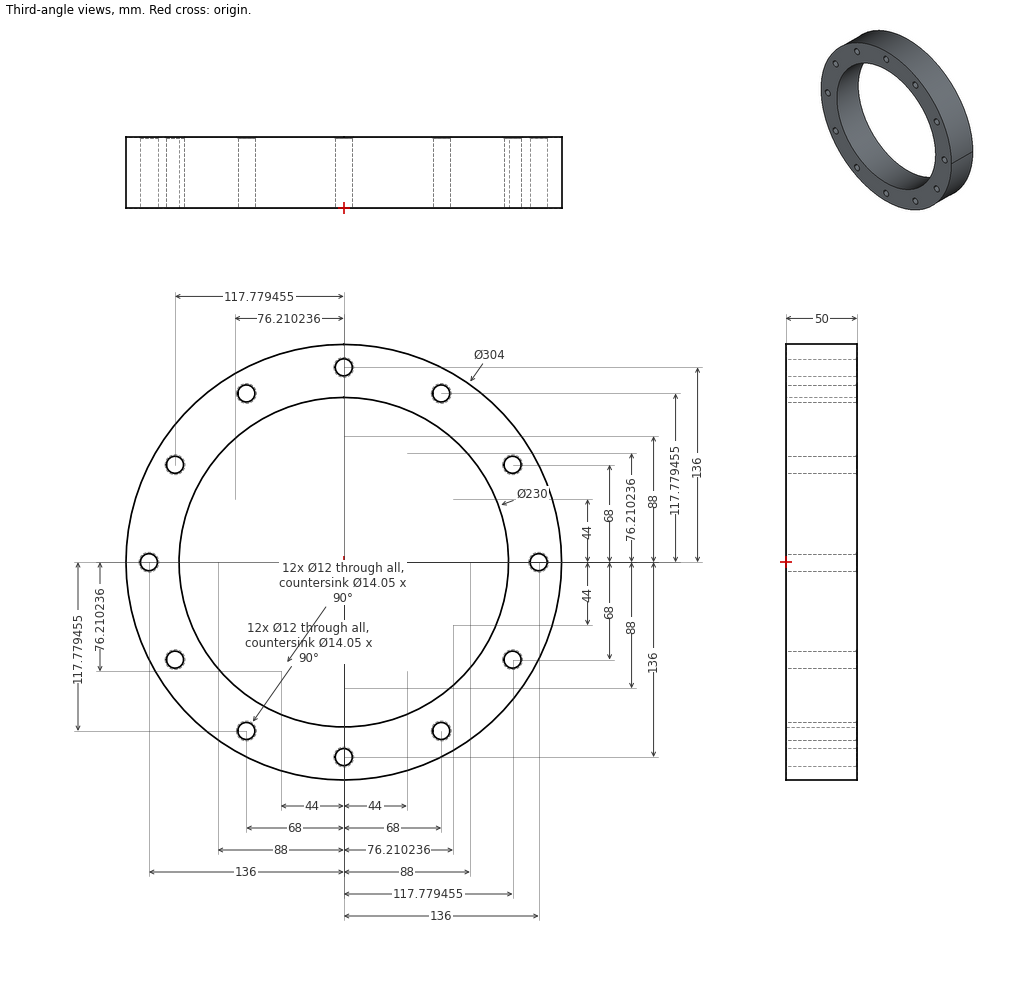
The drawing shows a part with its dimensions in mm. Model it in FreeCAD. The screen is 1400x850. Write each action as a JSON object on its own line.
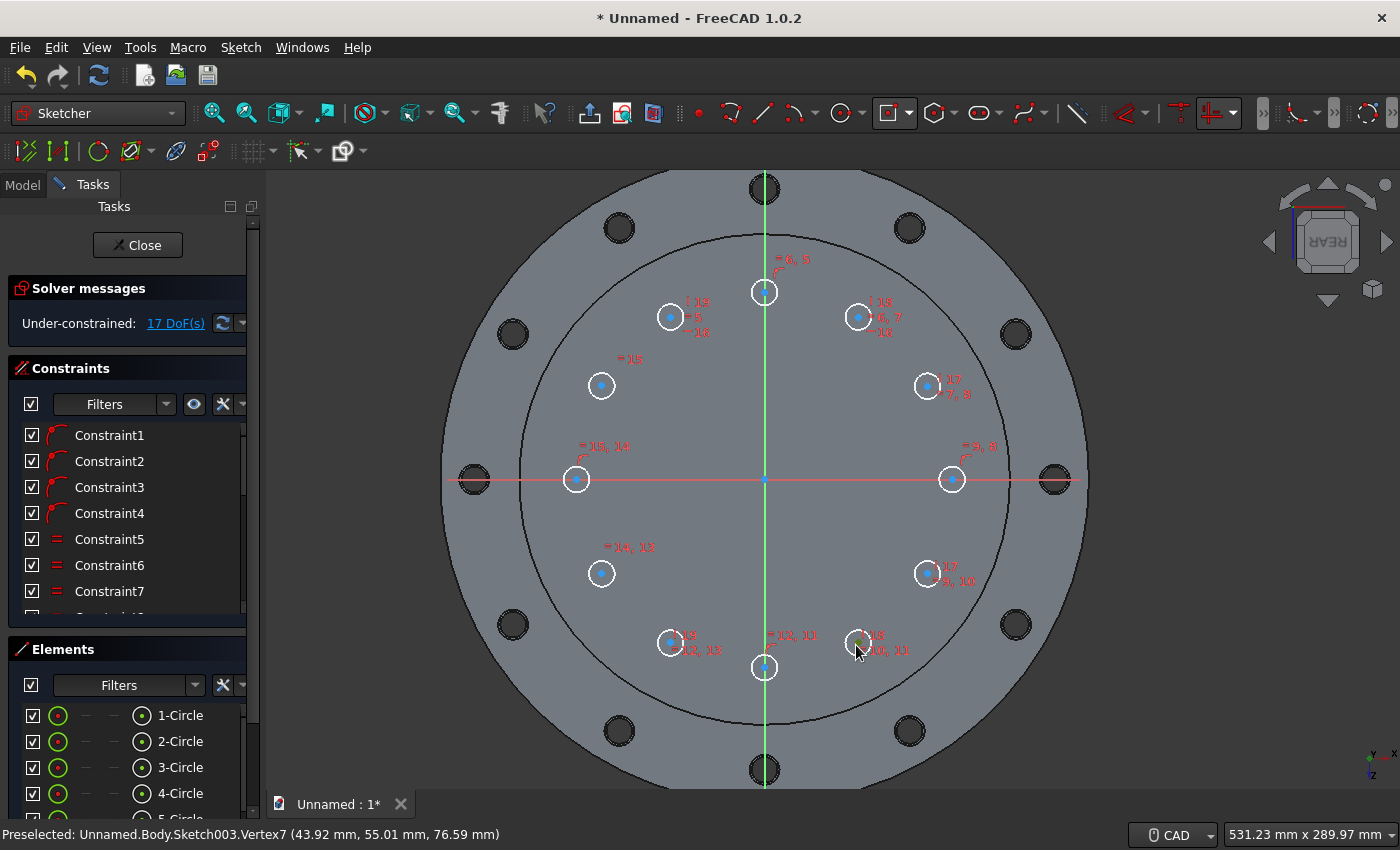
{"action": "left_click", "coordinate": [669, 645]}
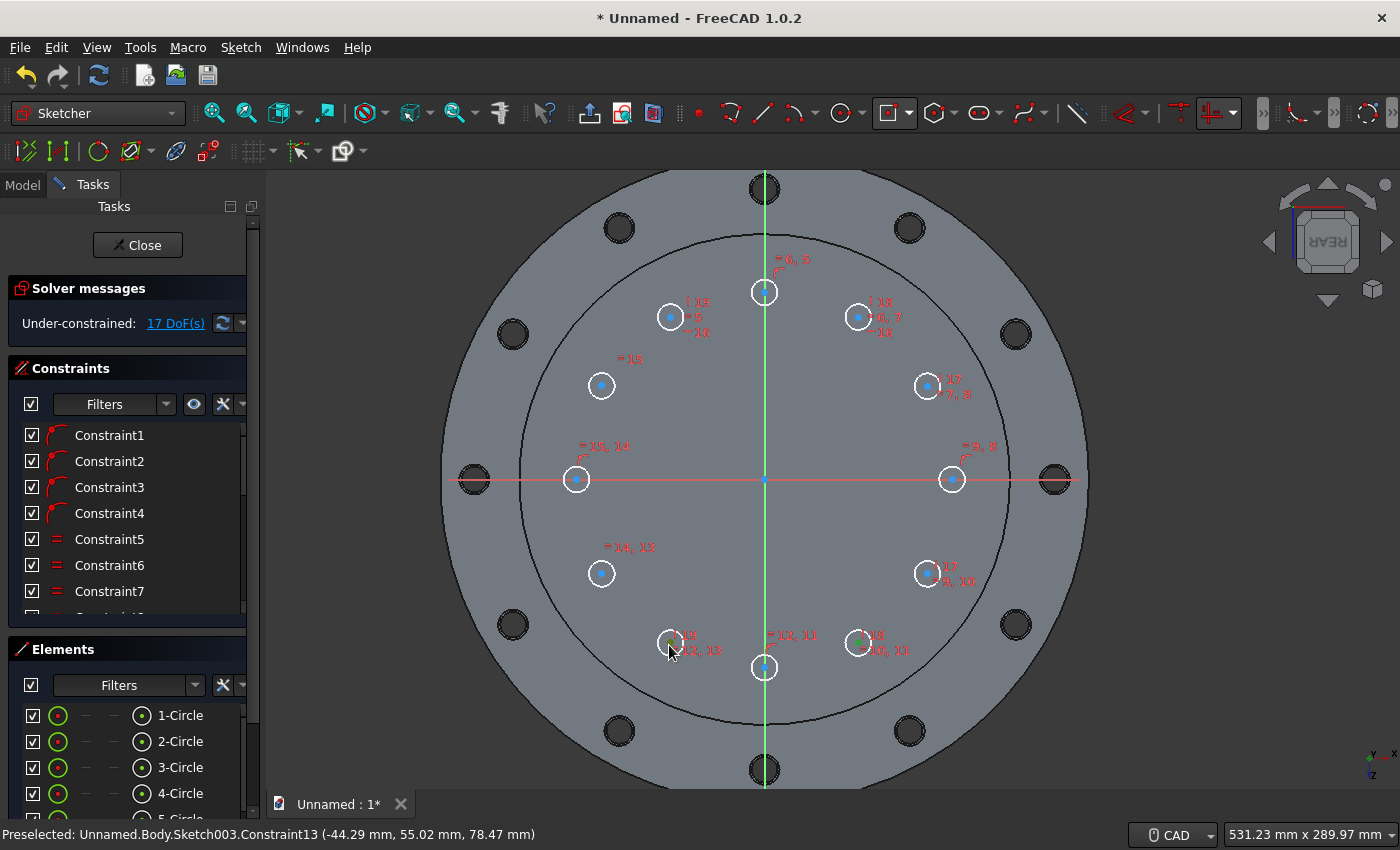
{"action": "key", "text": "h"}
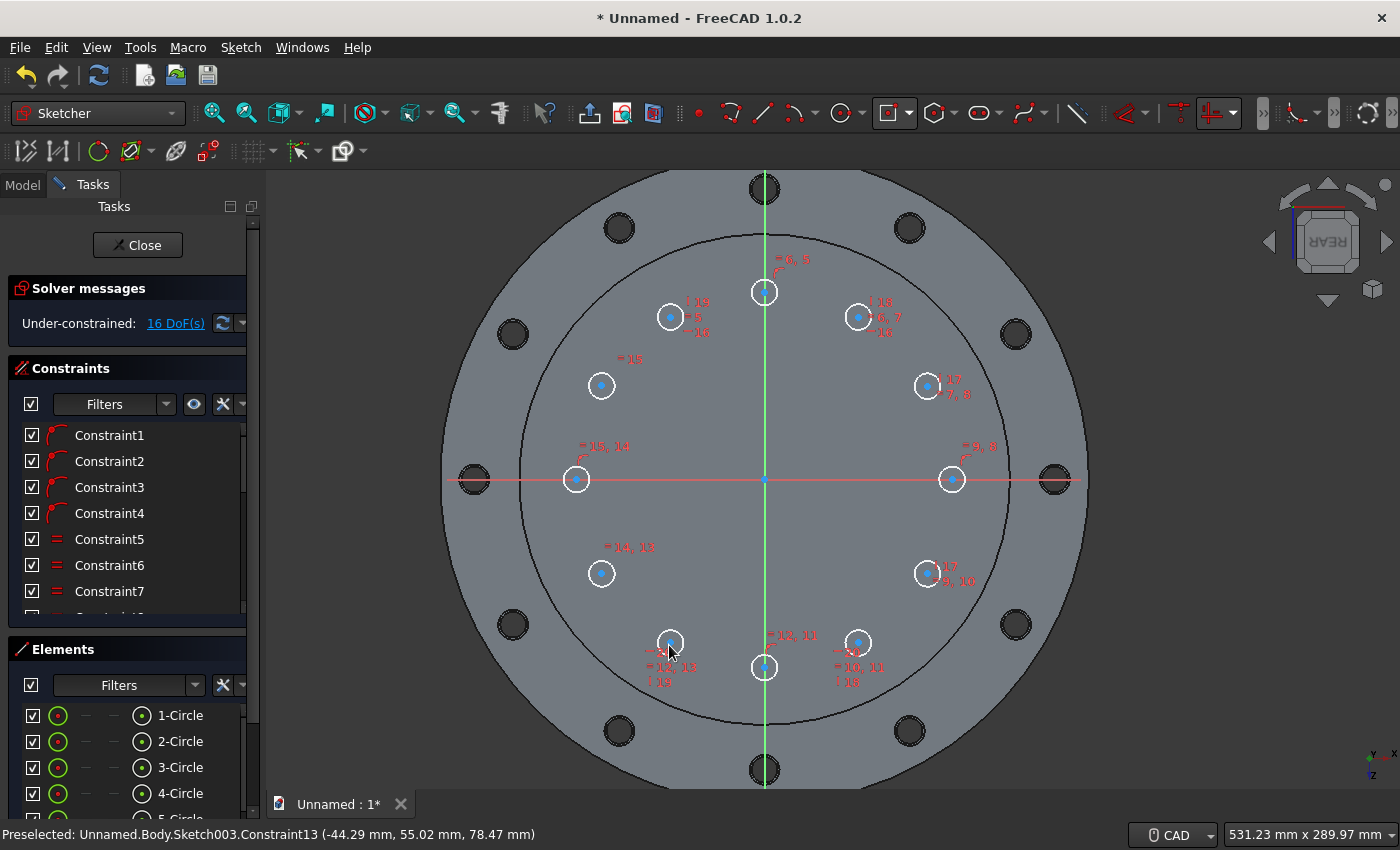
{"action": "left_click", "coordinate": [927, 574]}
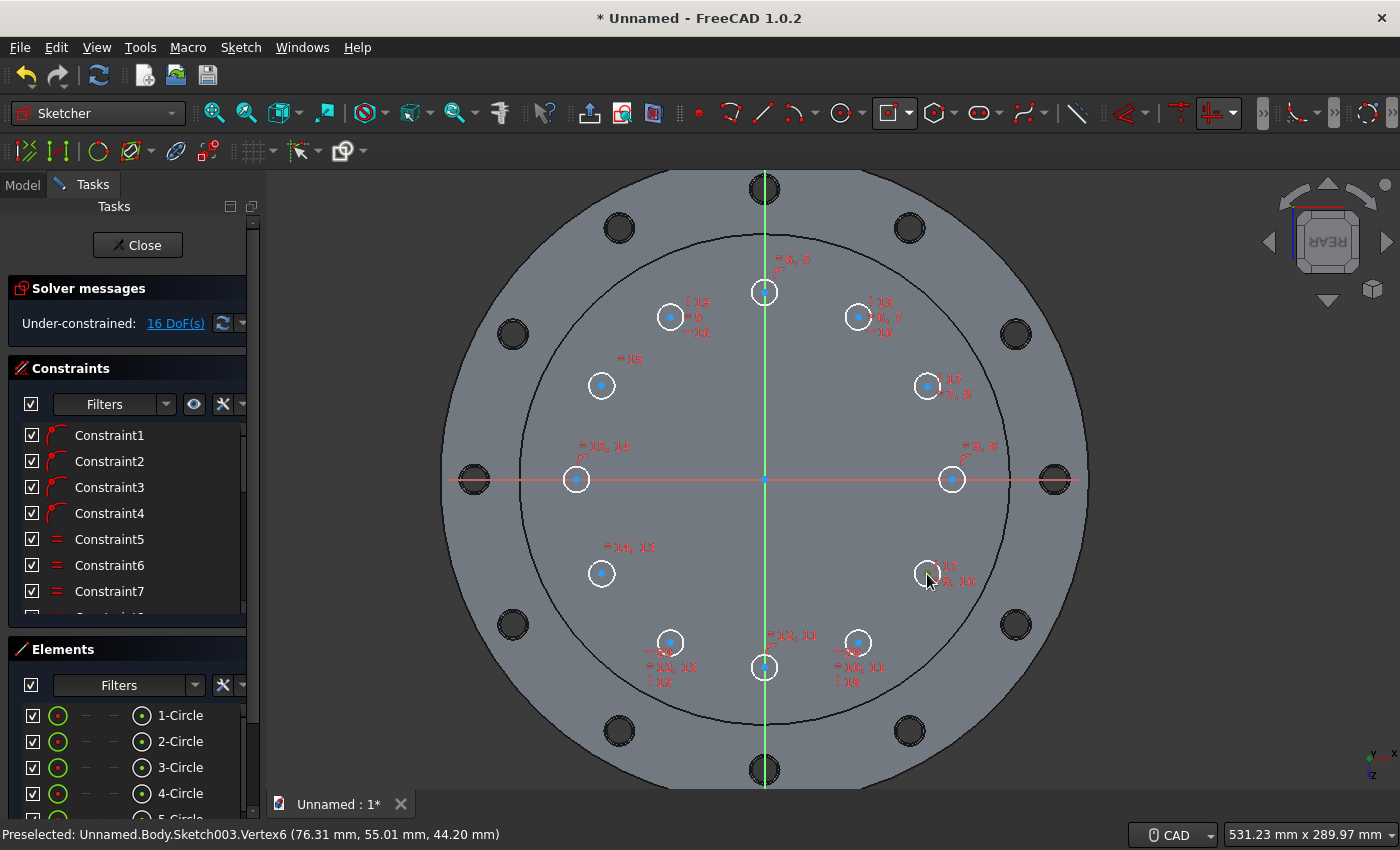
{"action": "left_click", "coordinate": [602, 574]}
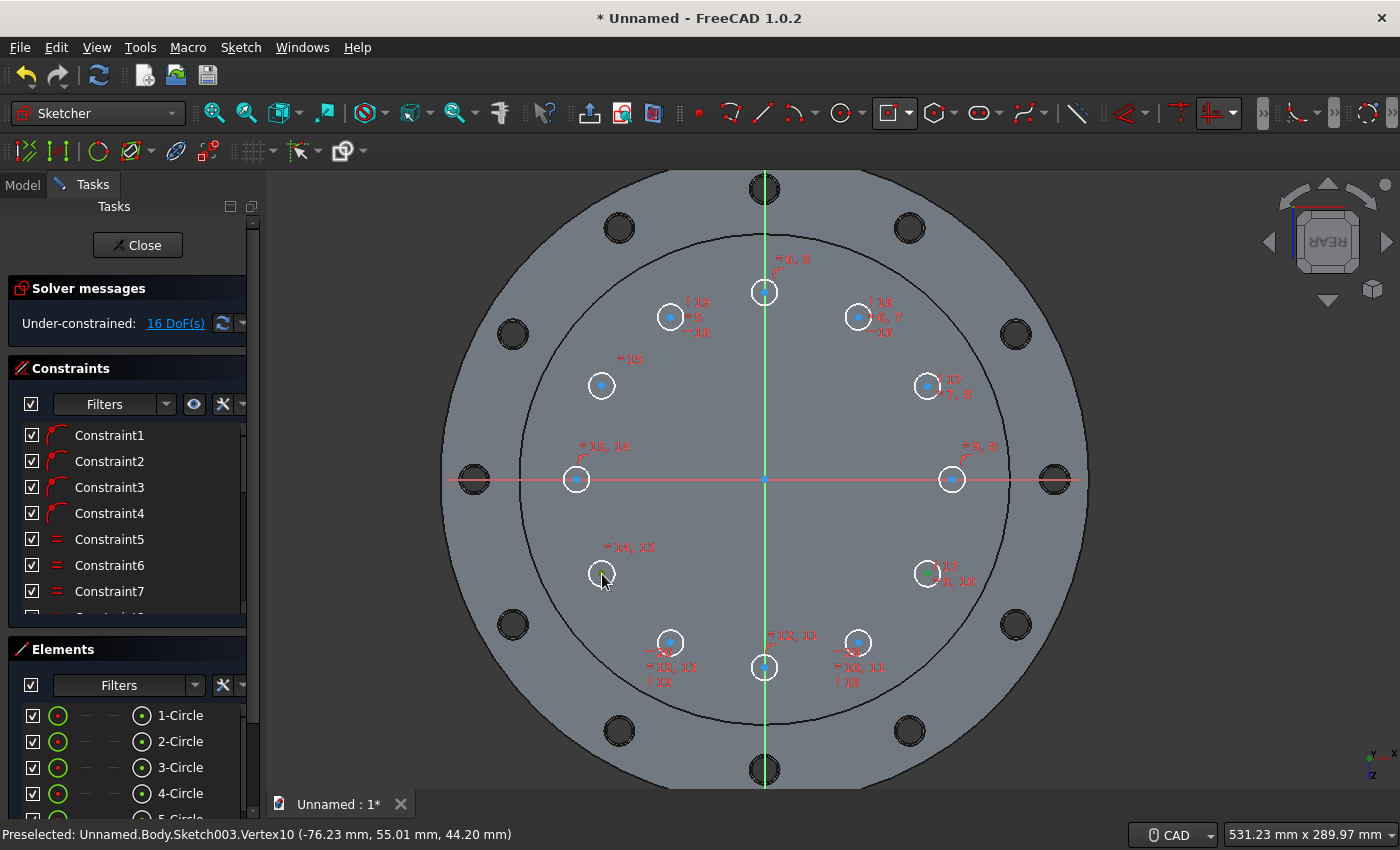
{"action": "key", "text": "h"}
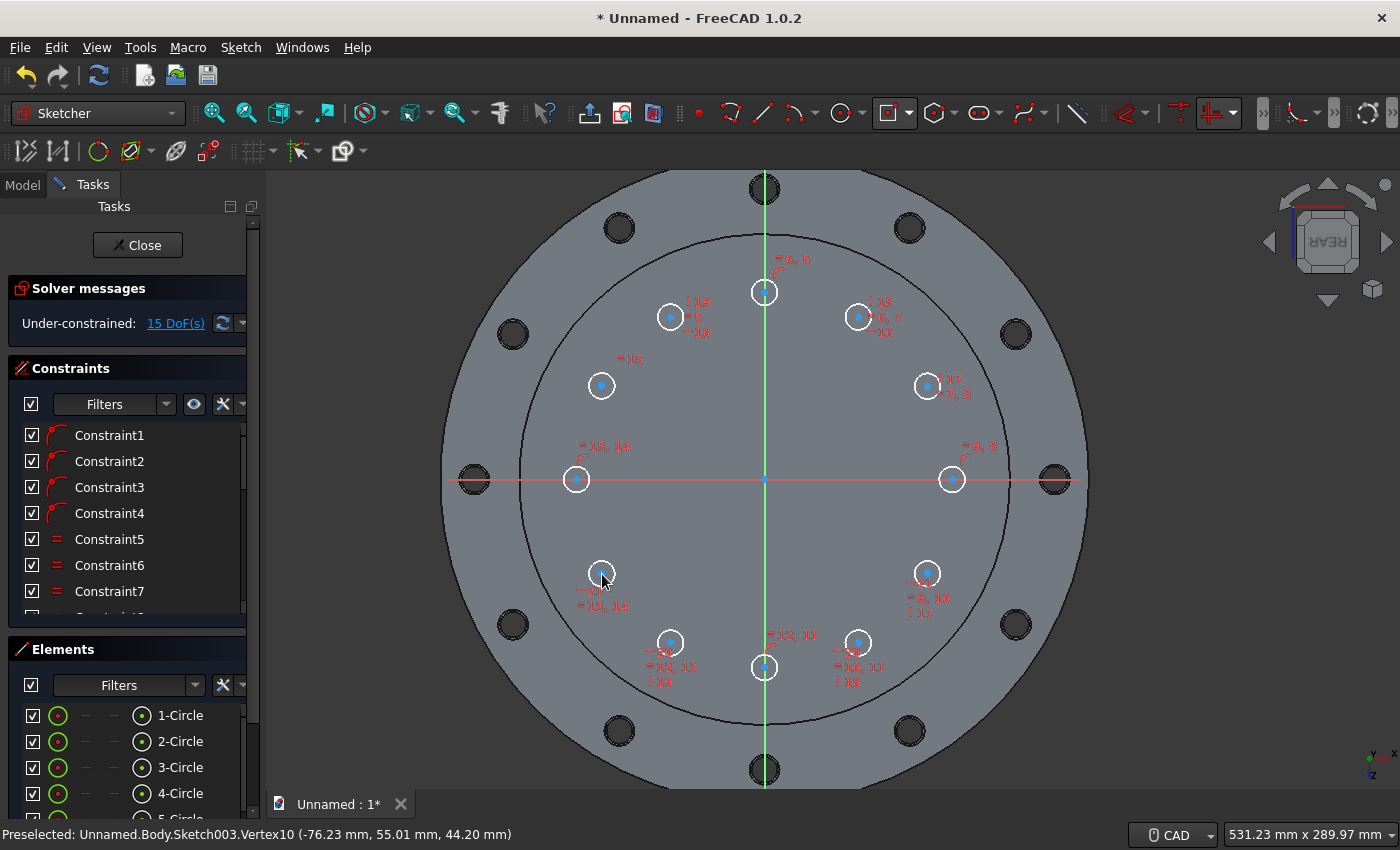
{"action": "left_click", "coordinate": [602, 574]}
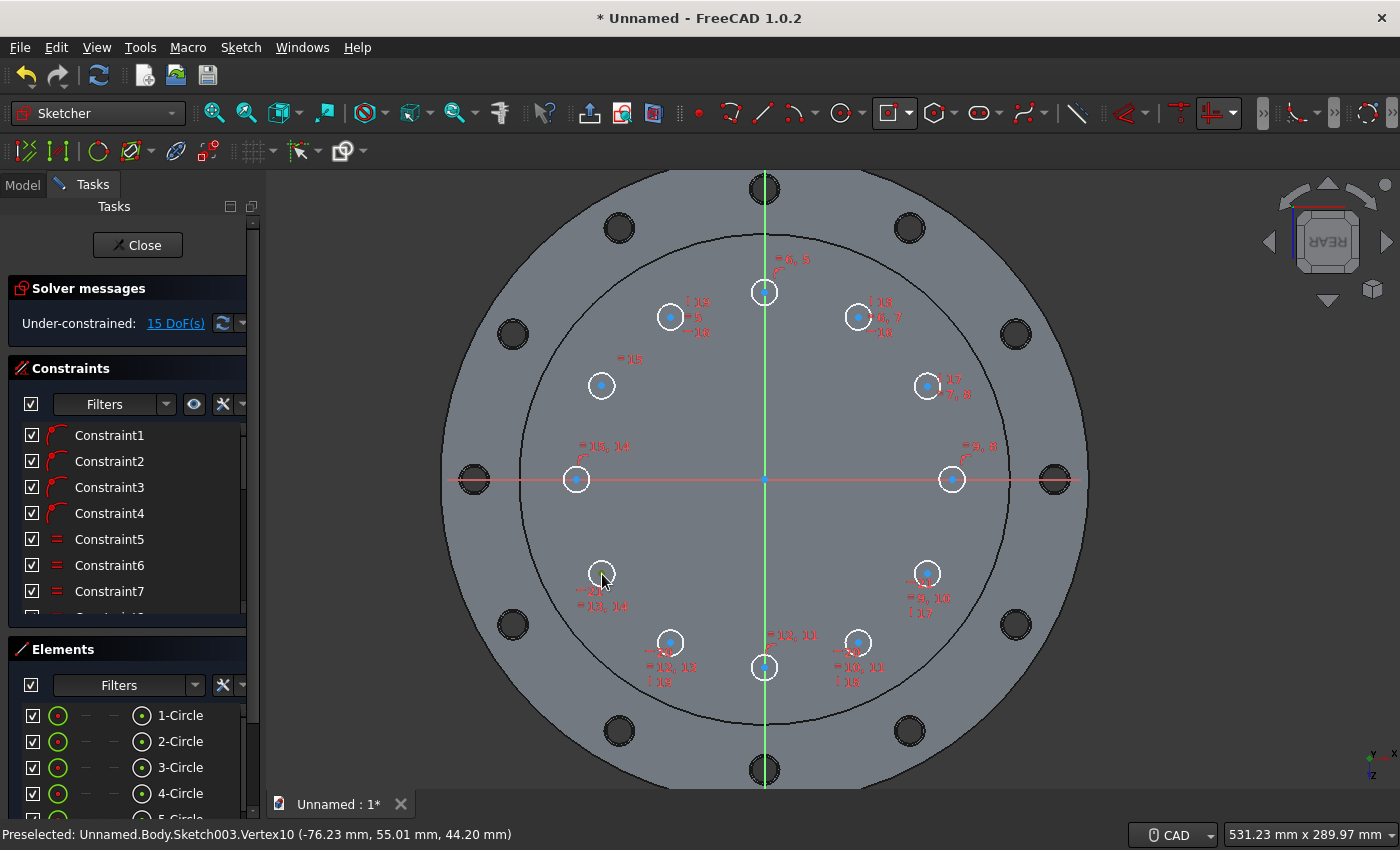
{"action": "left_click", "coordinate": [602, 386]}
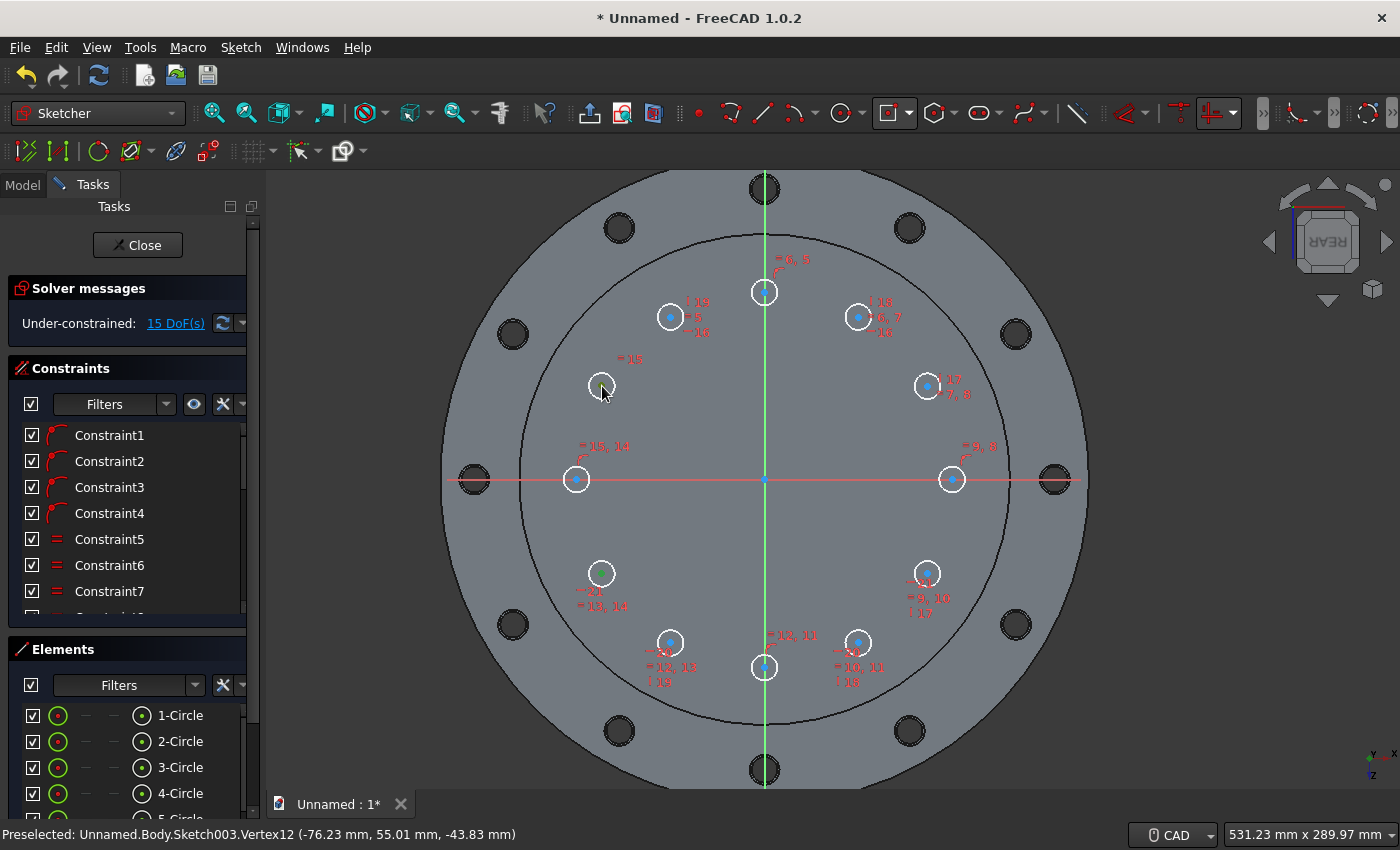
{"action": "left_click", "coordinate": [1236, 114]}